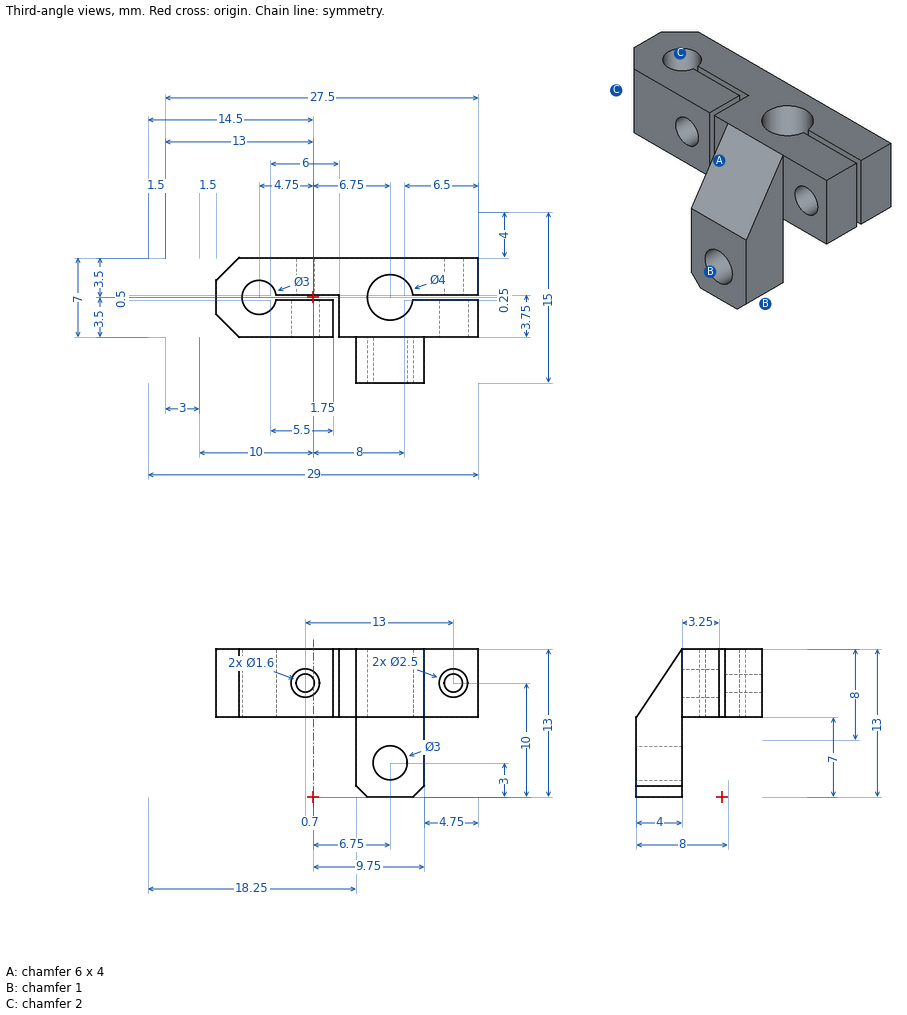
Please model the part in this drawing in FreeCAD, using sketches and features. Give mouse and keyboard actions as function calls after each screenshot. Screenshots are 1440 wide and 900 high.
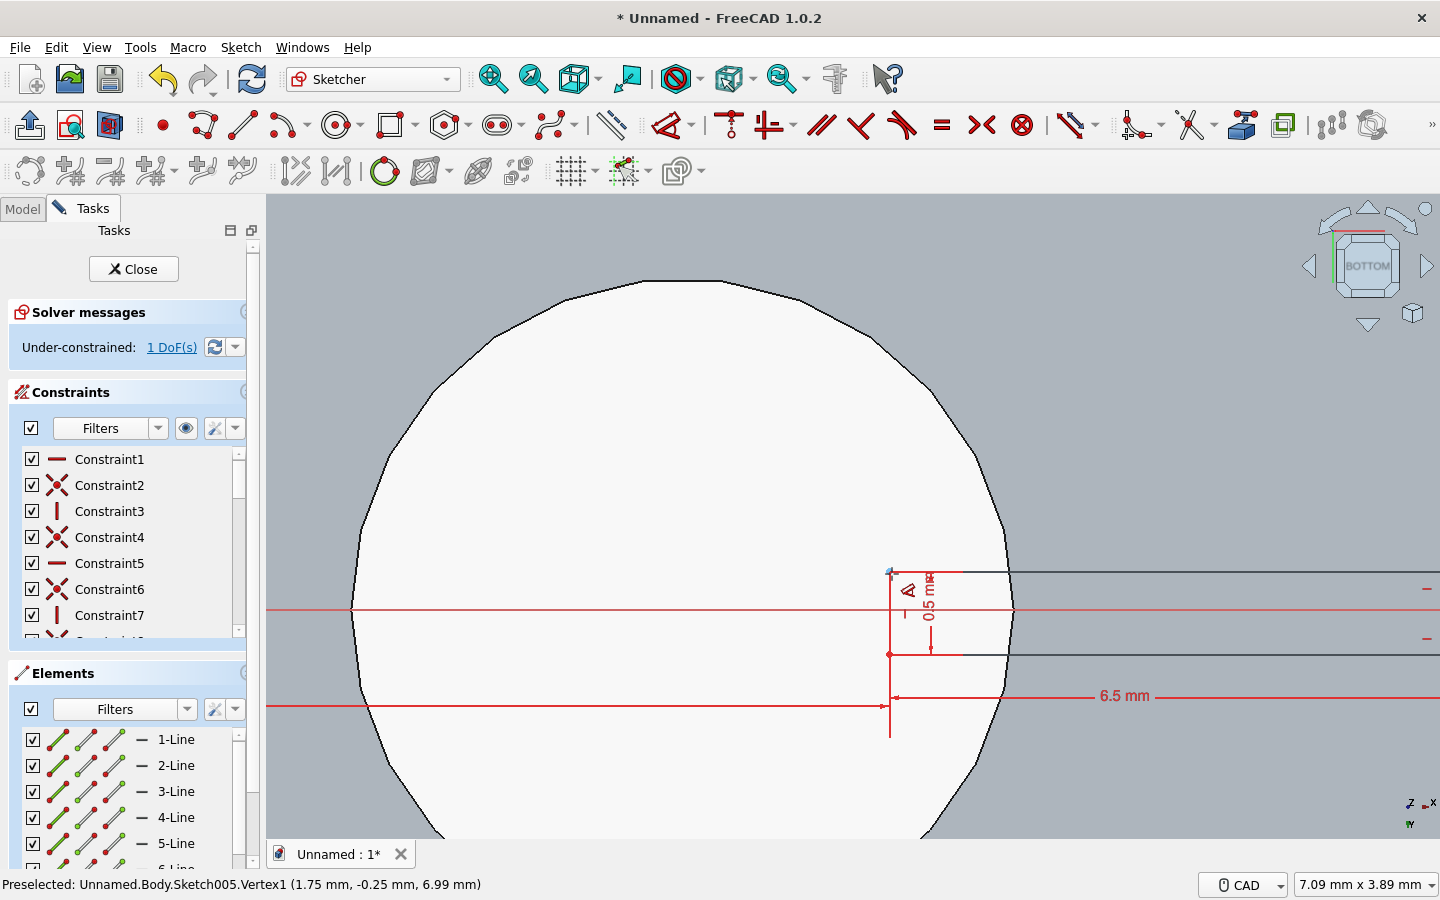
click(890, 572)
click(1020, 591)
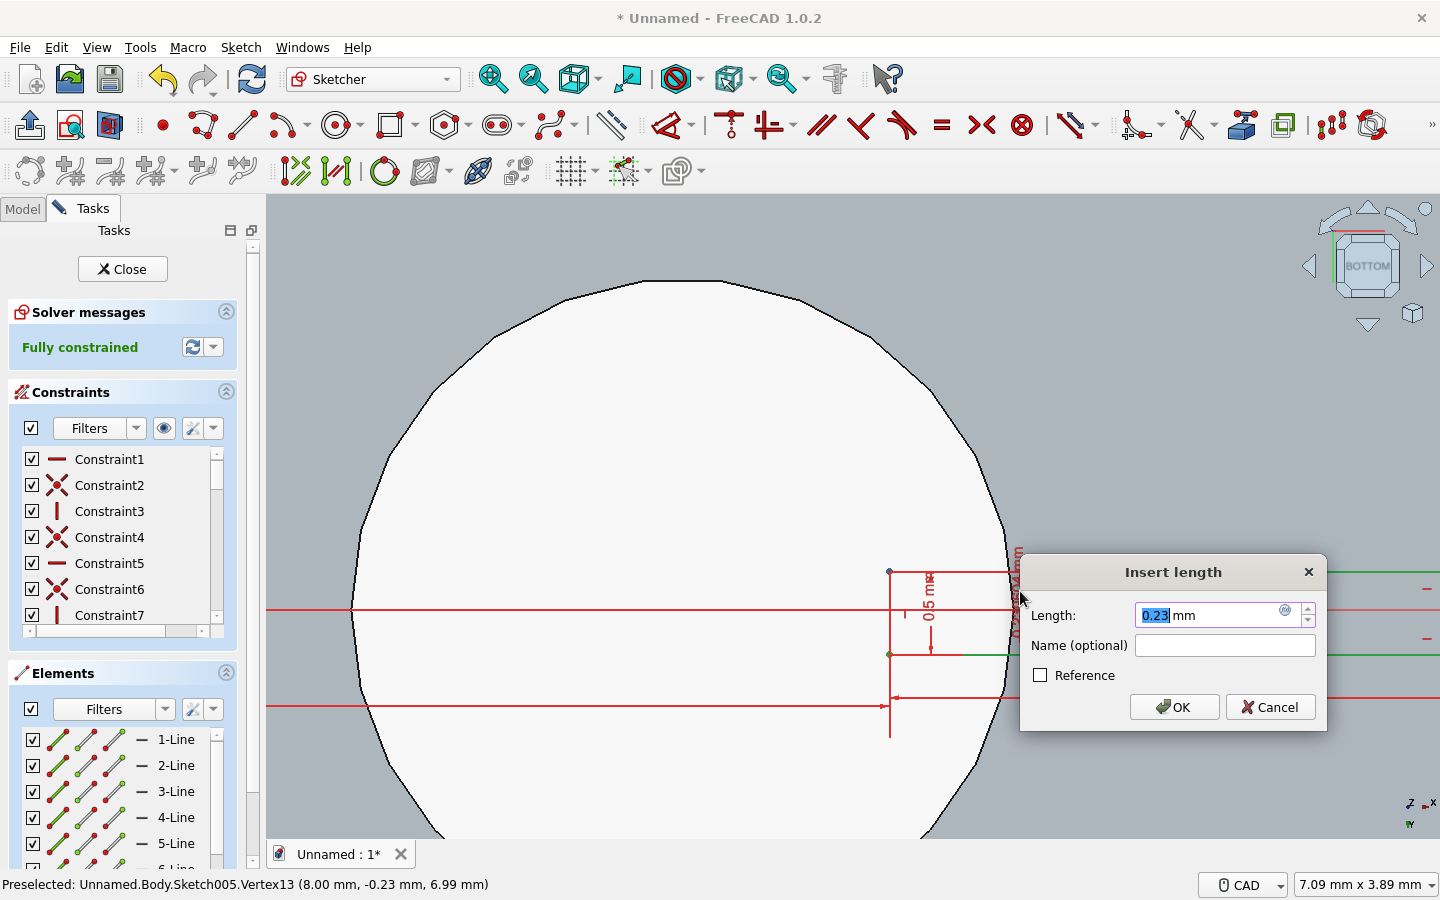
text(0.25)
key(Return)
key(Escape)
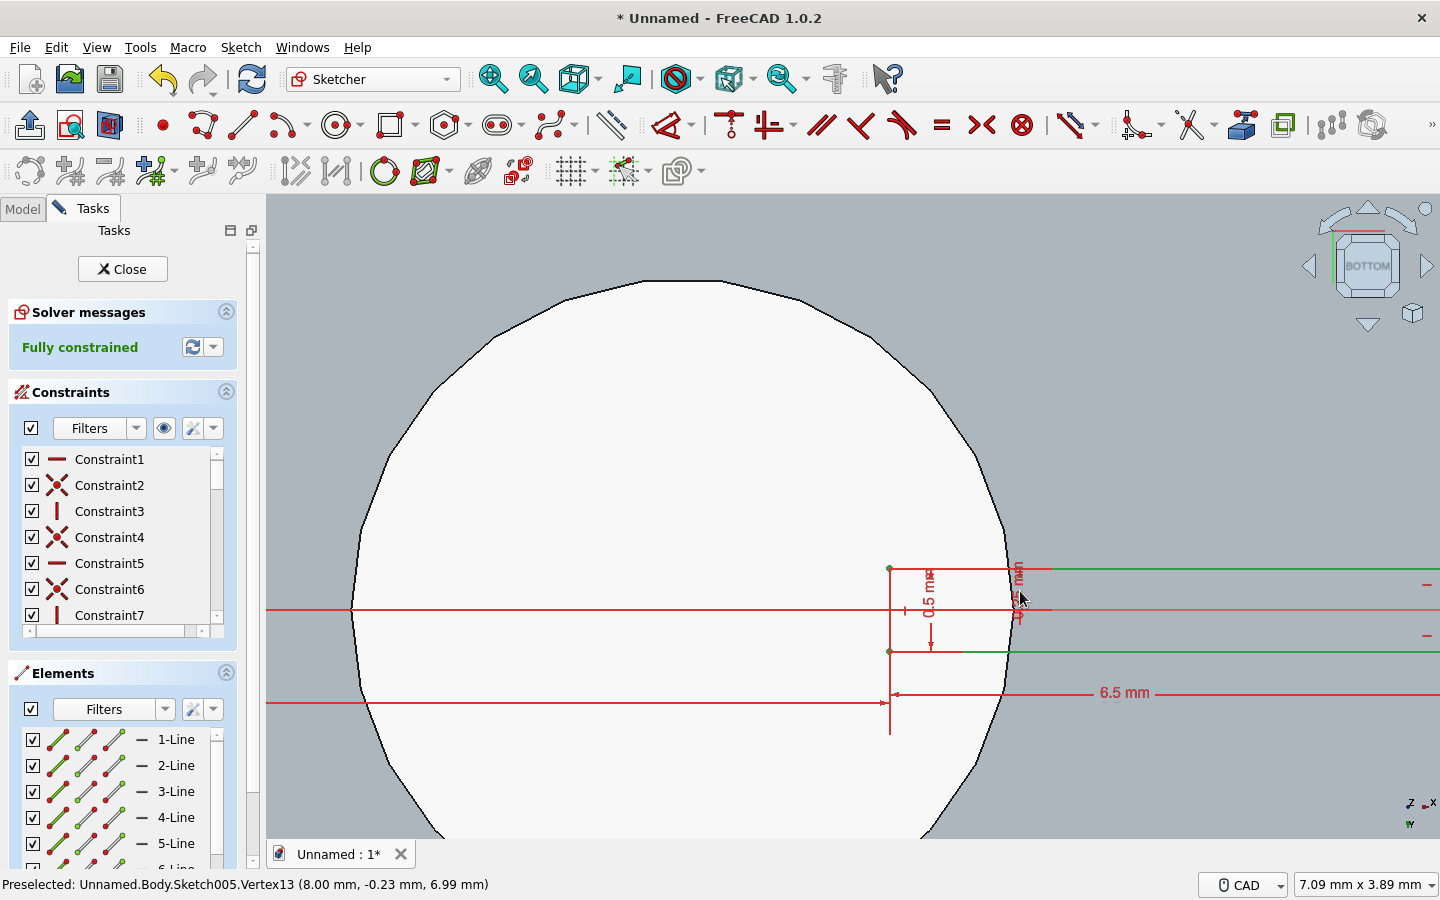
click(123, 269)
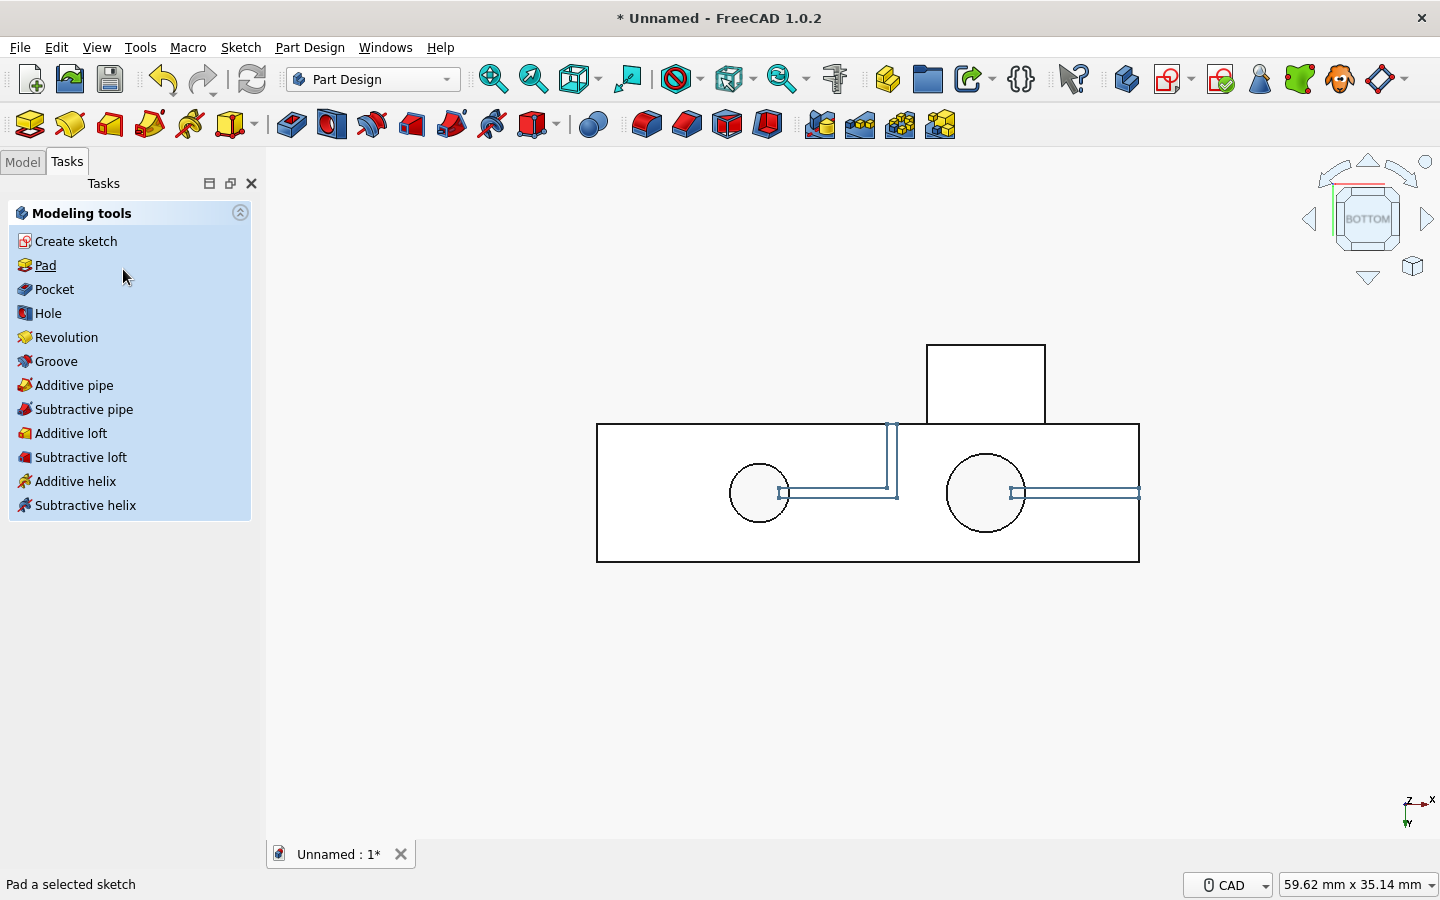
click(292, 124)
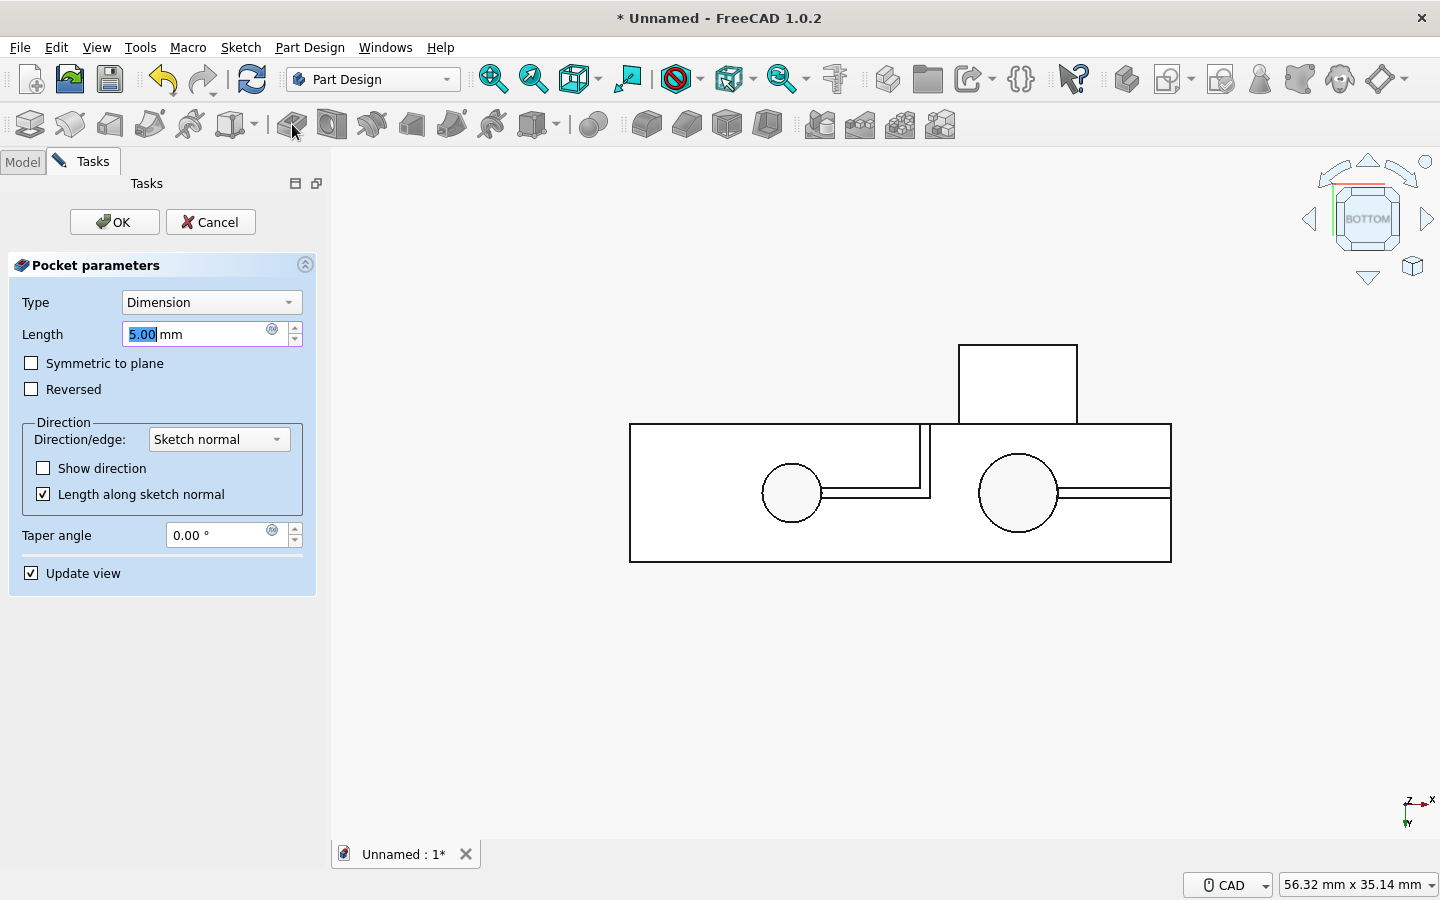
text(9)
key(Tab)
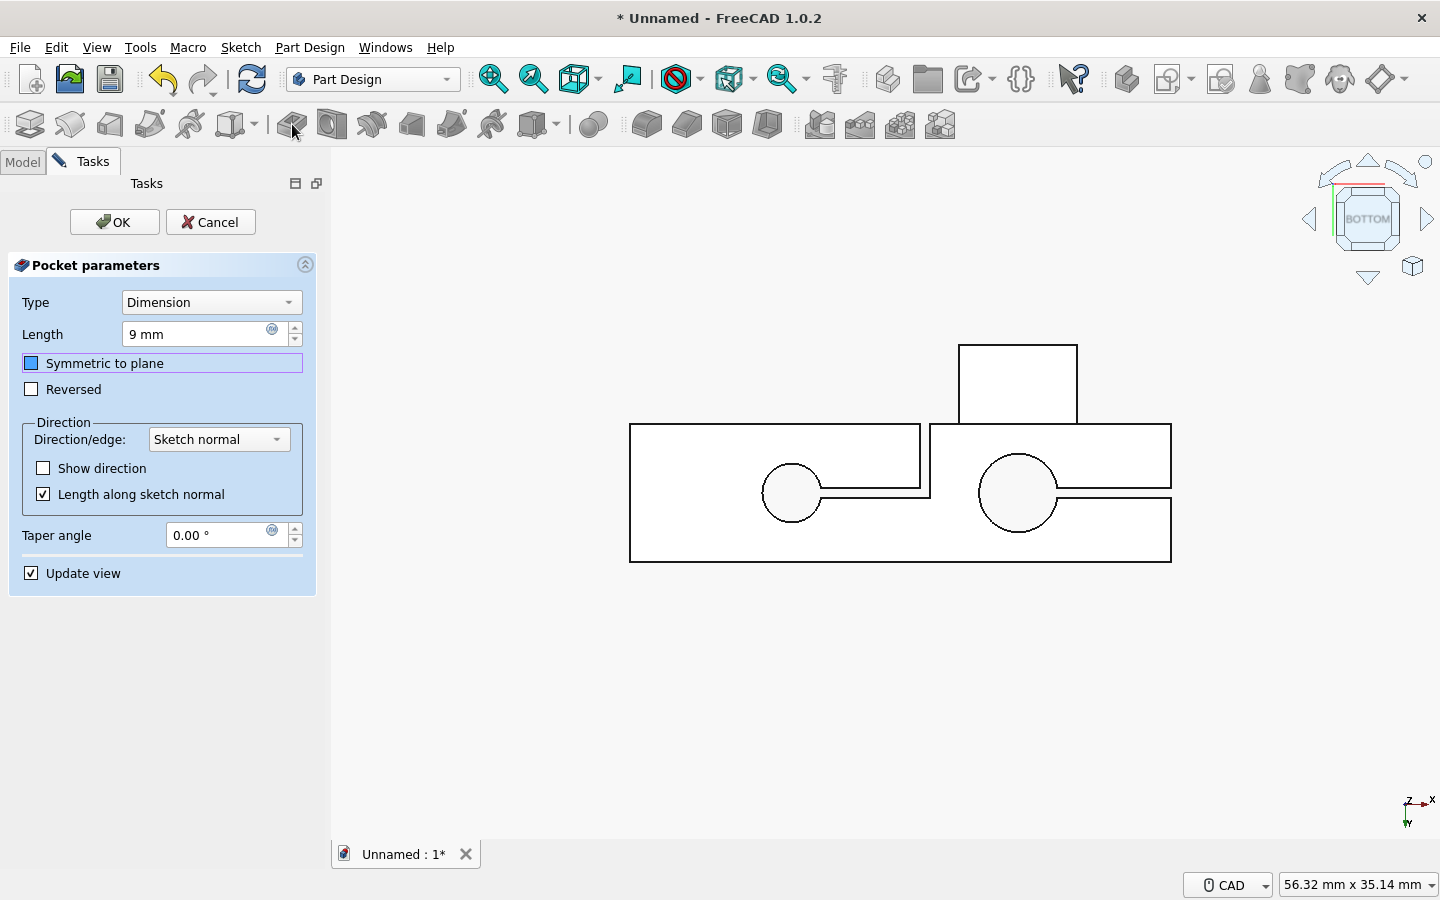
click(115, 222)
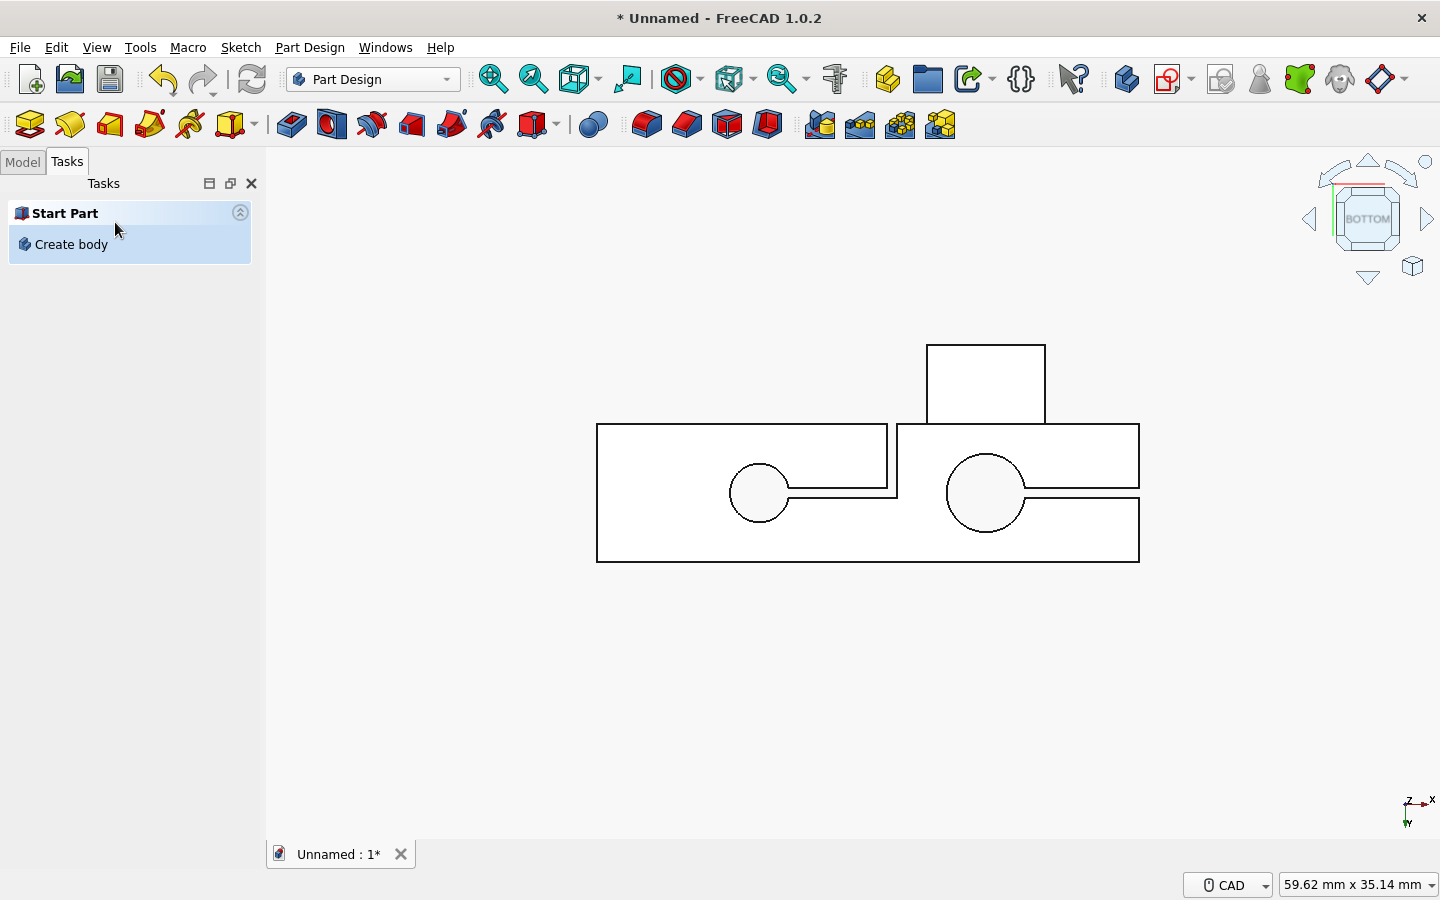
key(0)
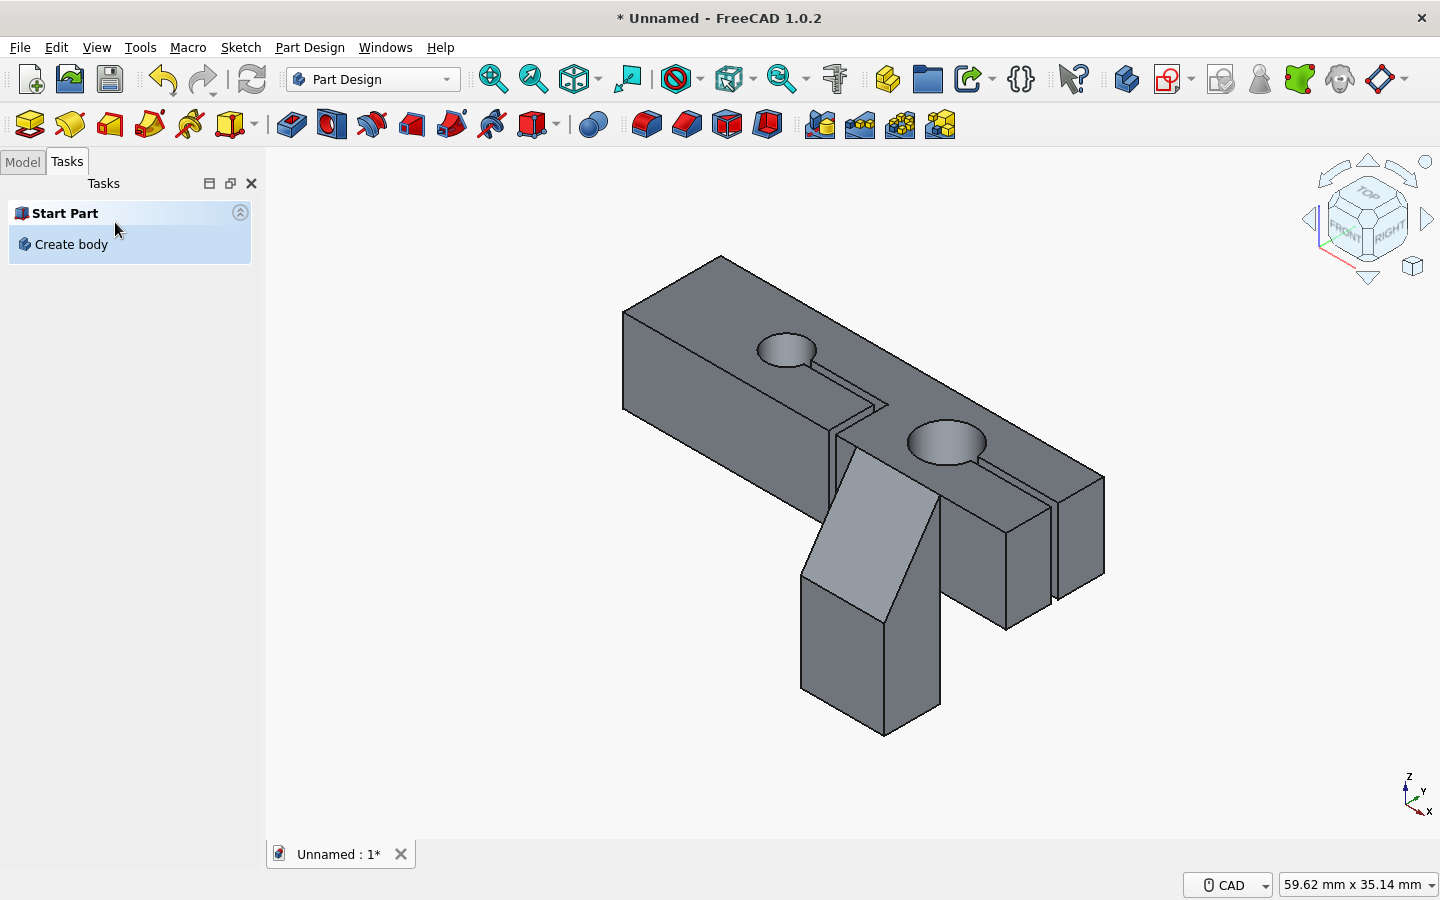
click(785, 453)